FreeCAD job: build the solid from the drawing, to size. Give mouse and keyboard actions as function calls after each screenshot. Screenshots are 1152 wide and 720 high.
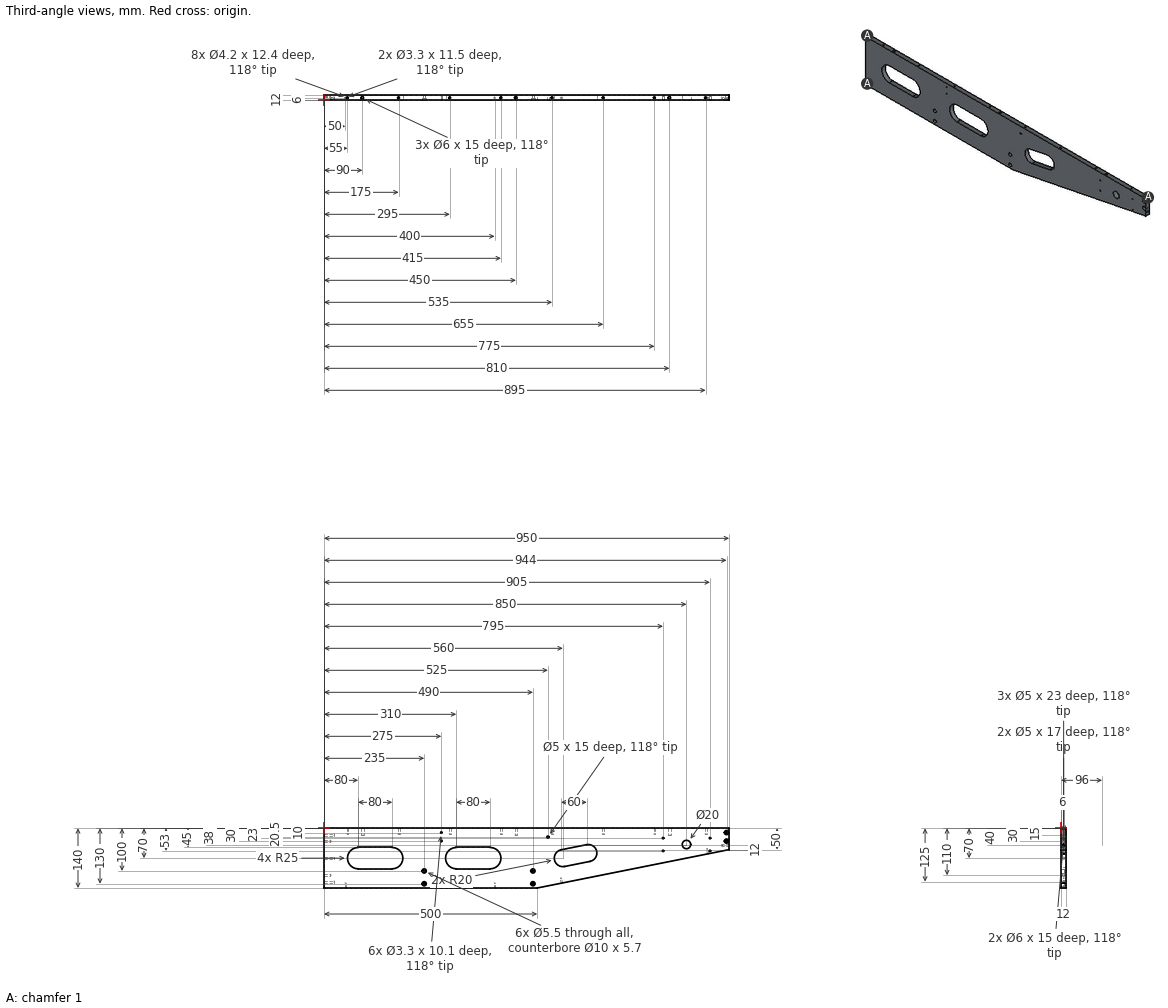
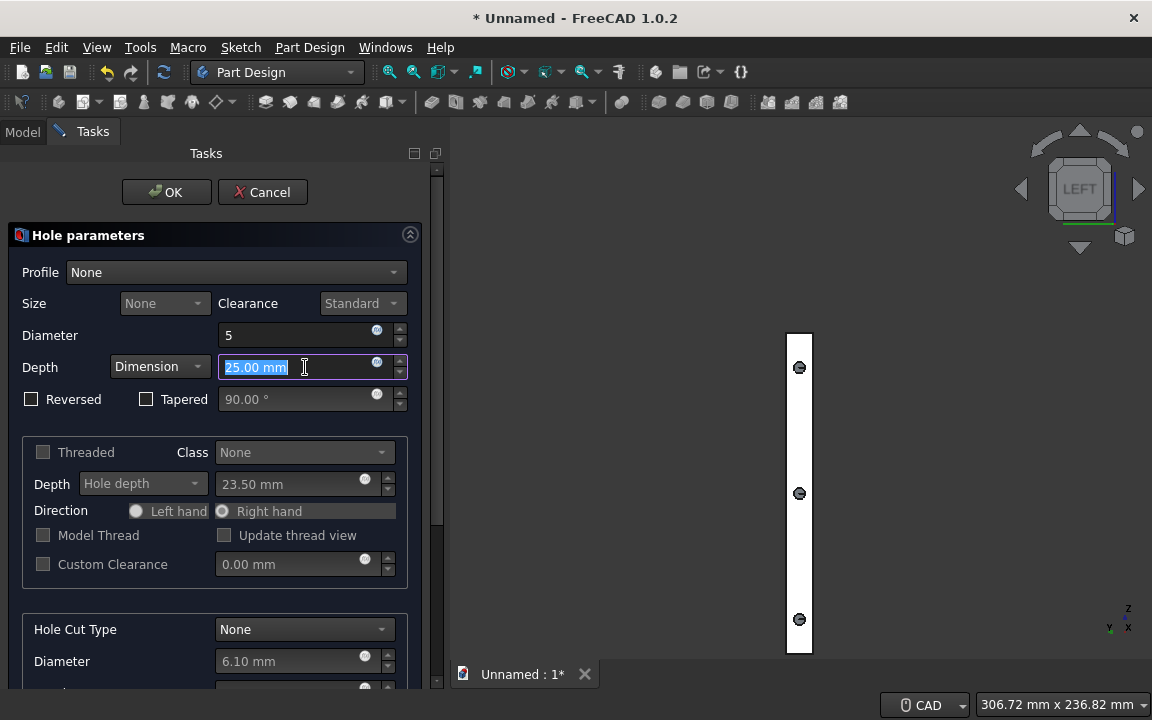
text(23)
key(Tab)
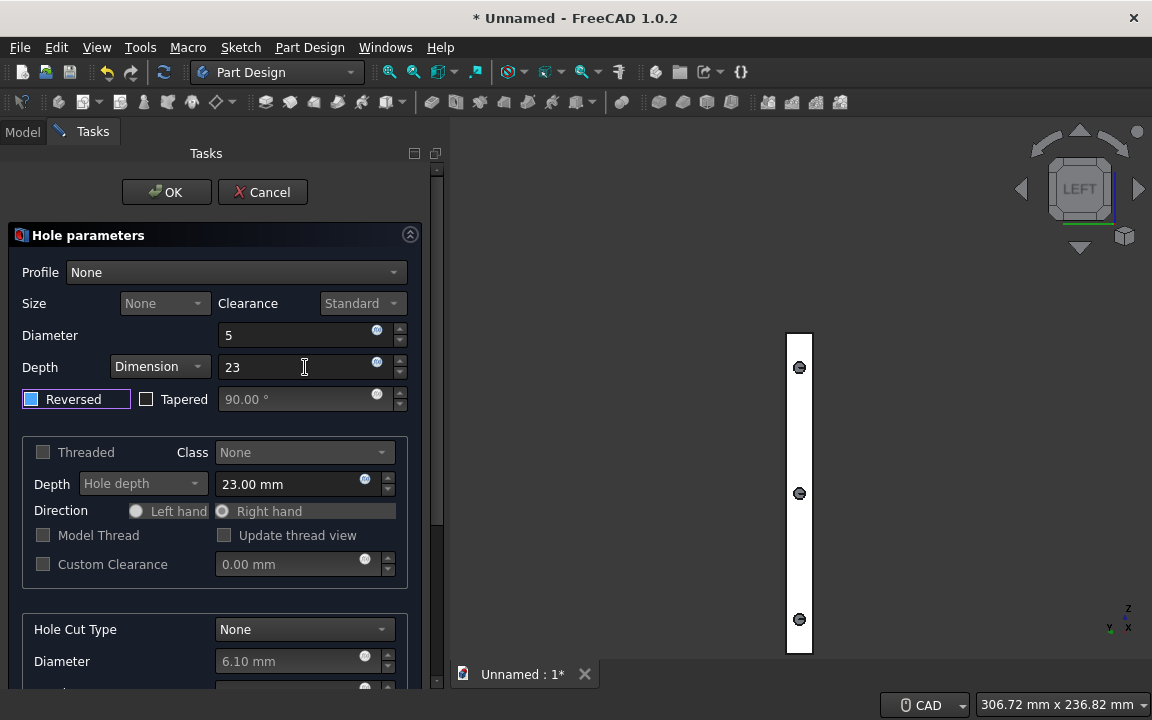
click(167, 192)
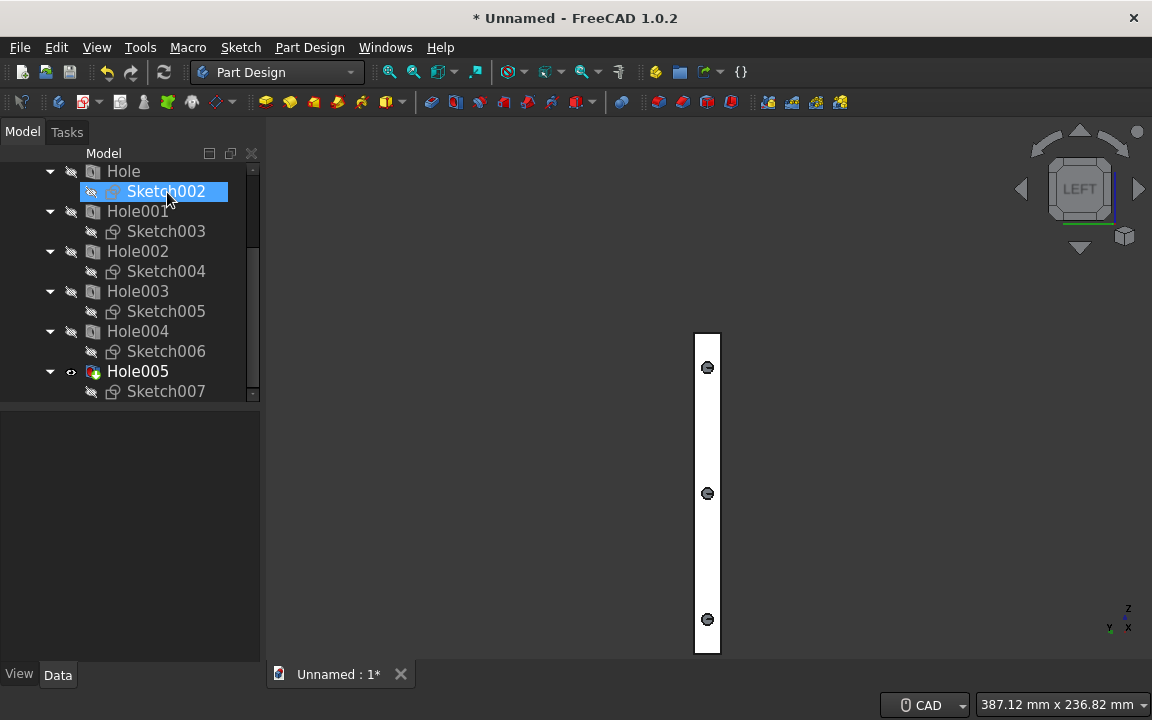
click(707, 401)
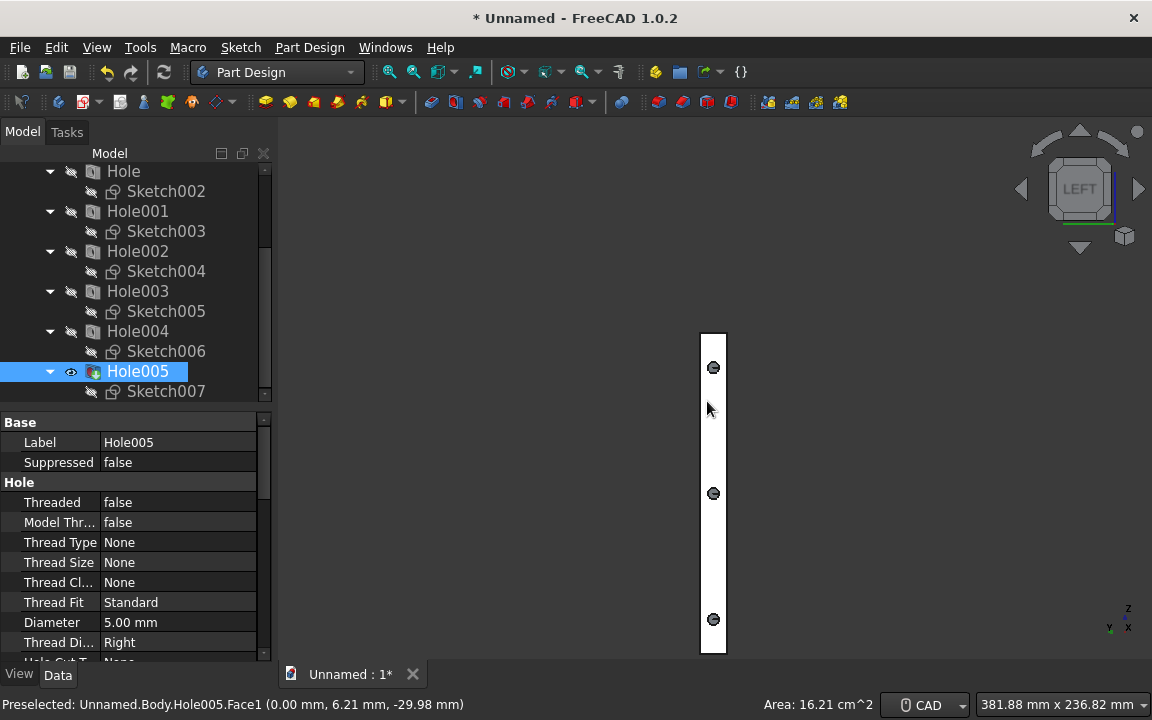
click(84, 102)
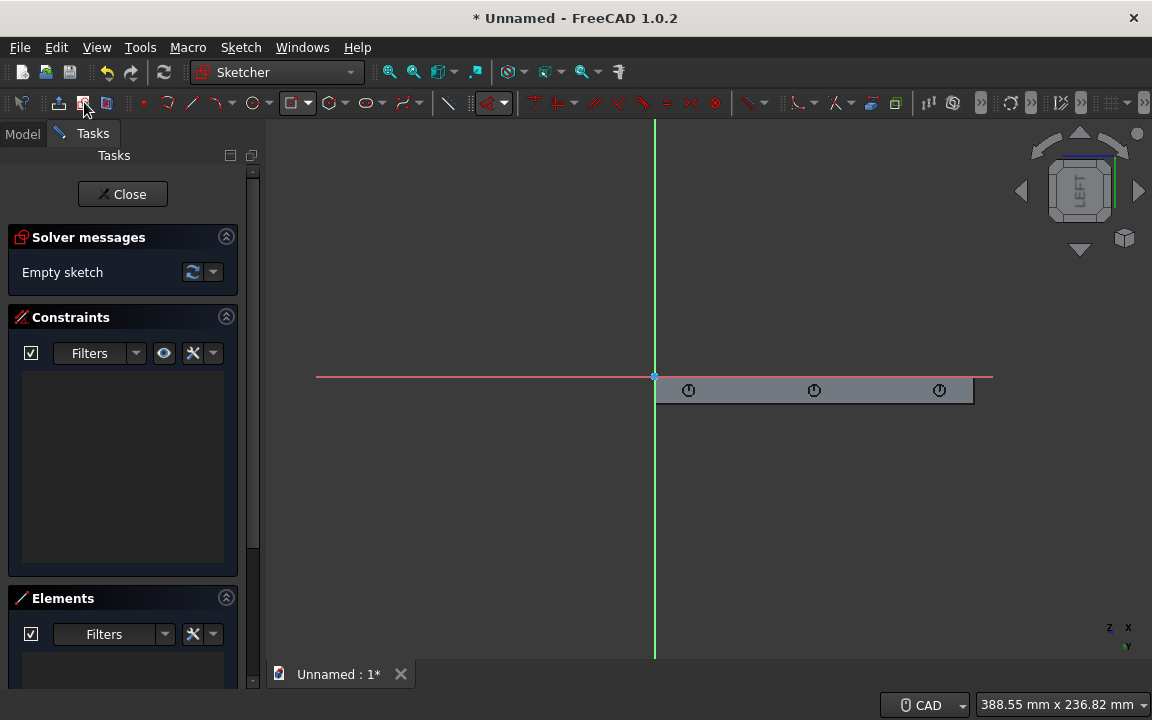
scroll(957, 385, up, 3)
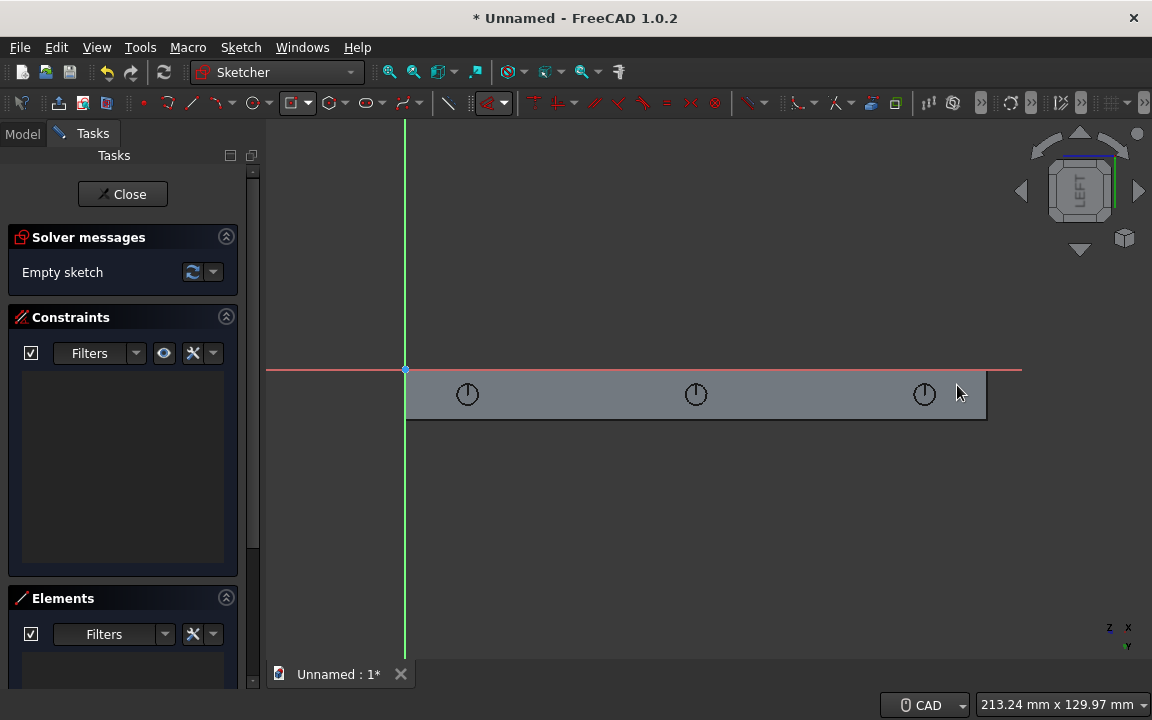
key(g)
key(c)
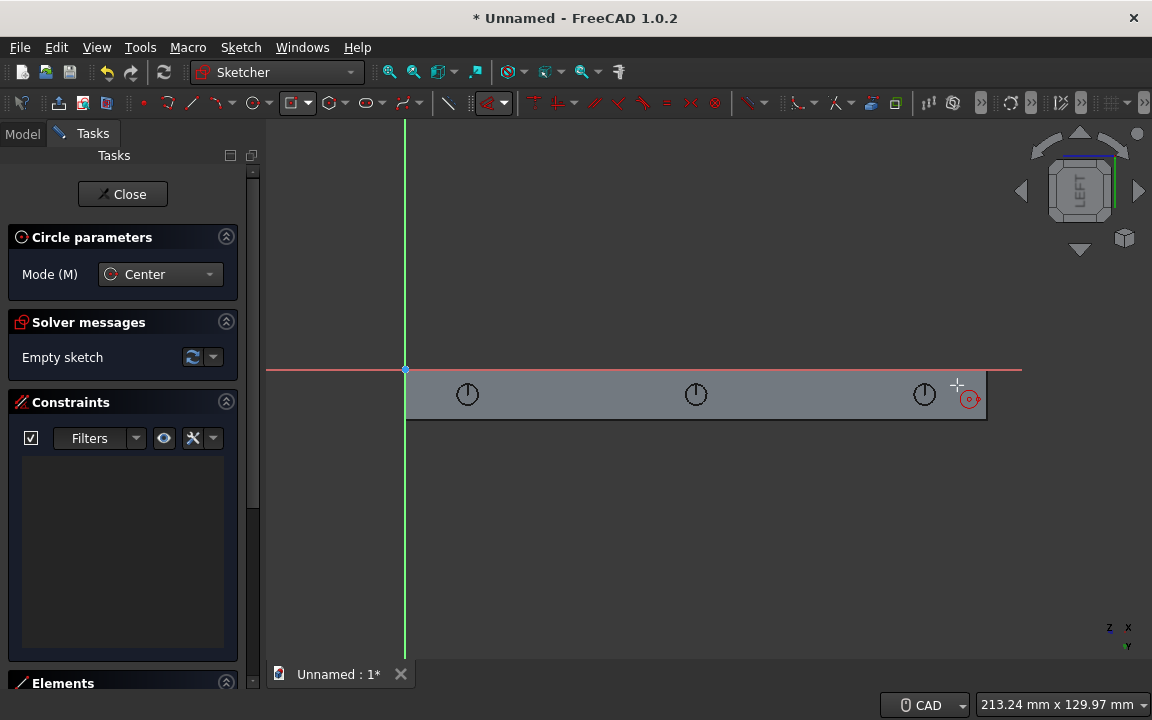
scroll(530, 395, up, 3)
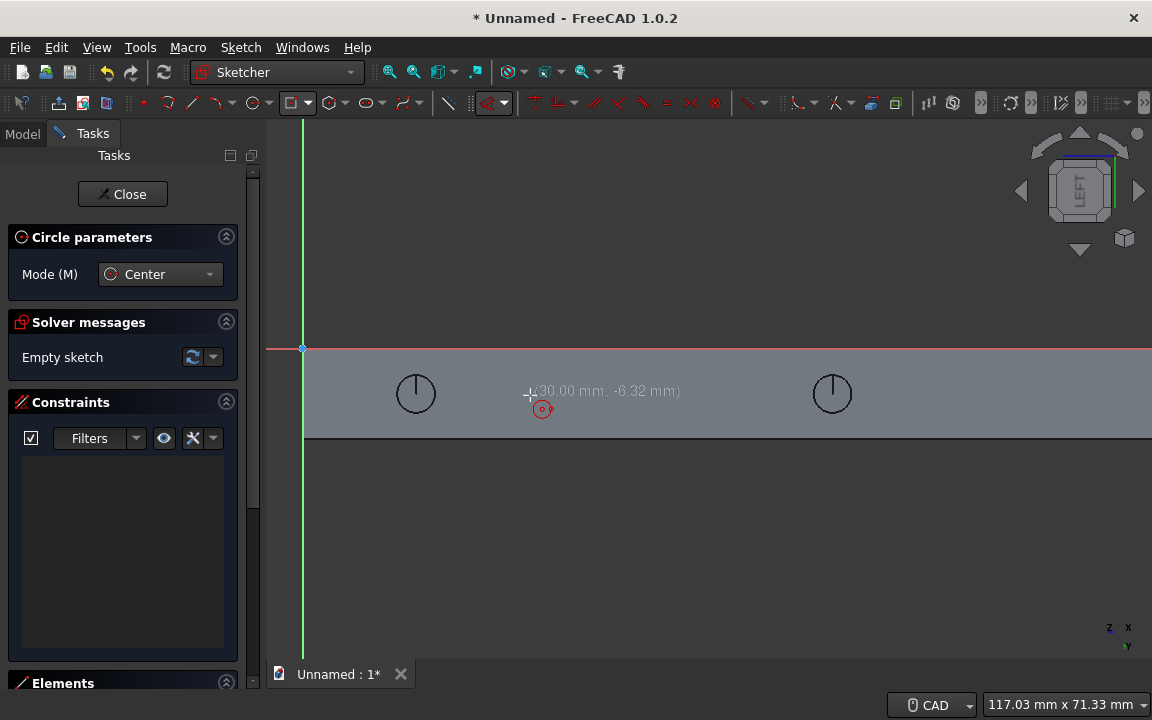
click(530, 394)
move(546, 378)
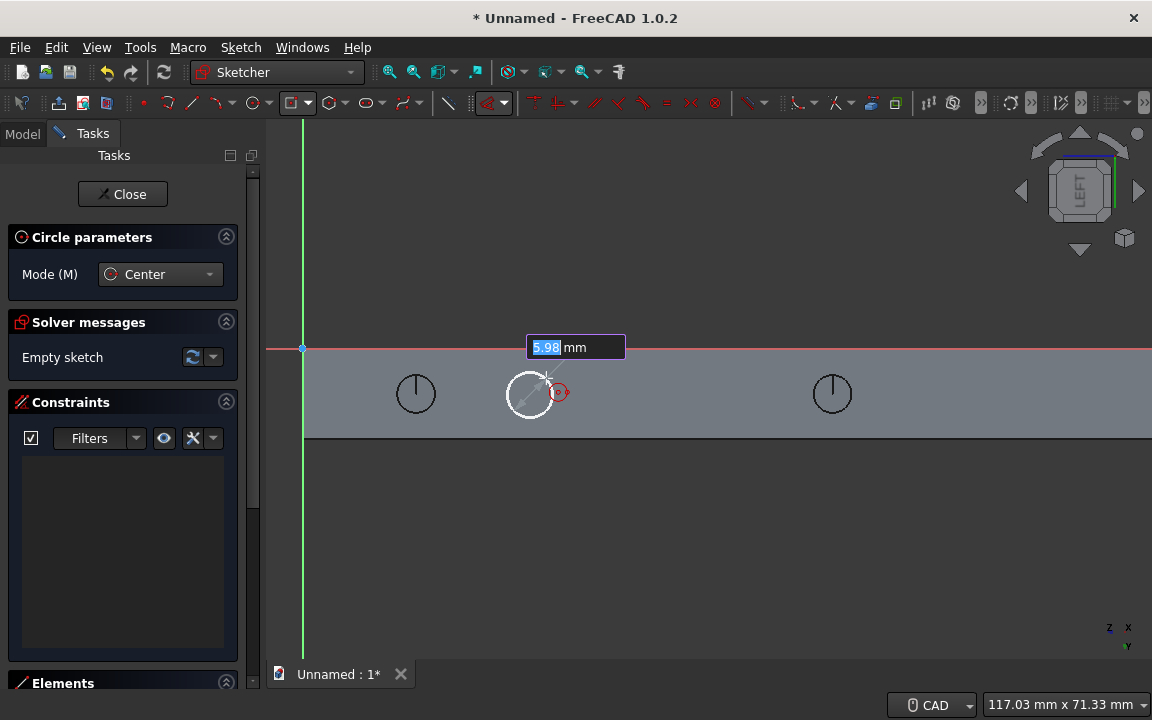
text(6)
key(Return)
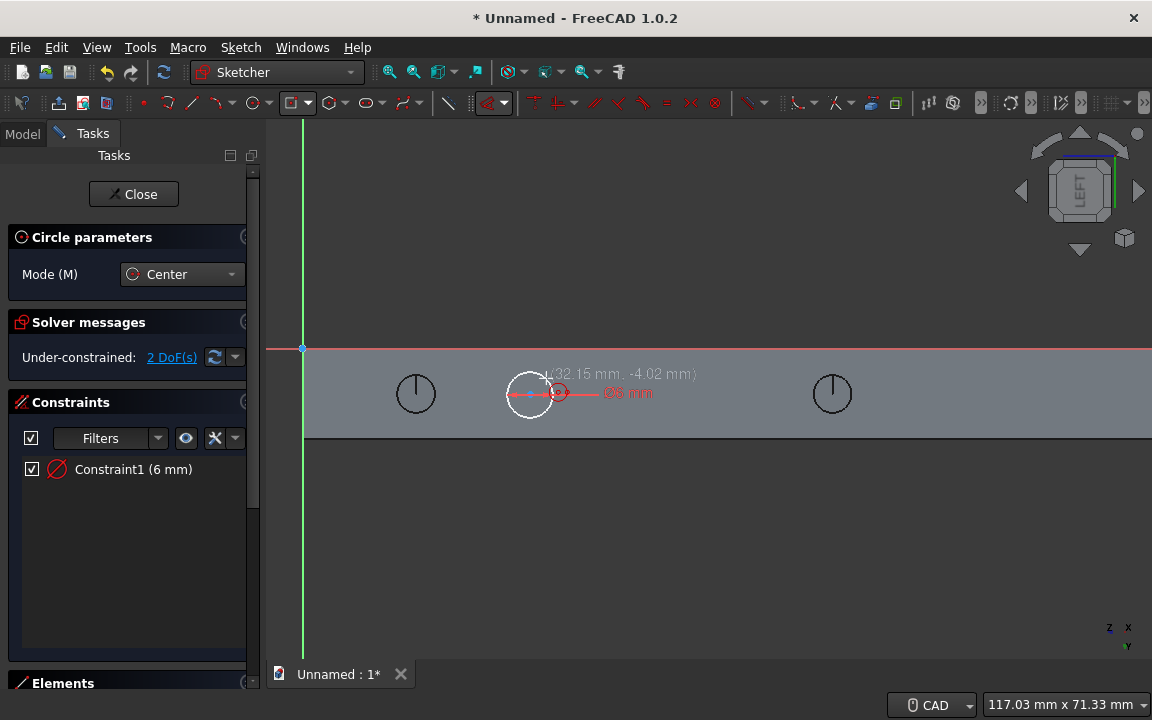
scroll(531, 397, down, 3)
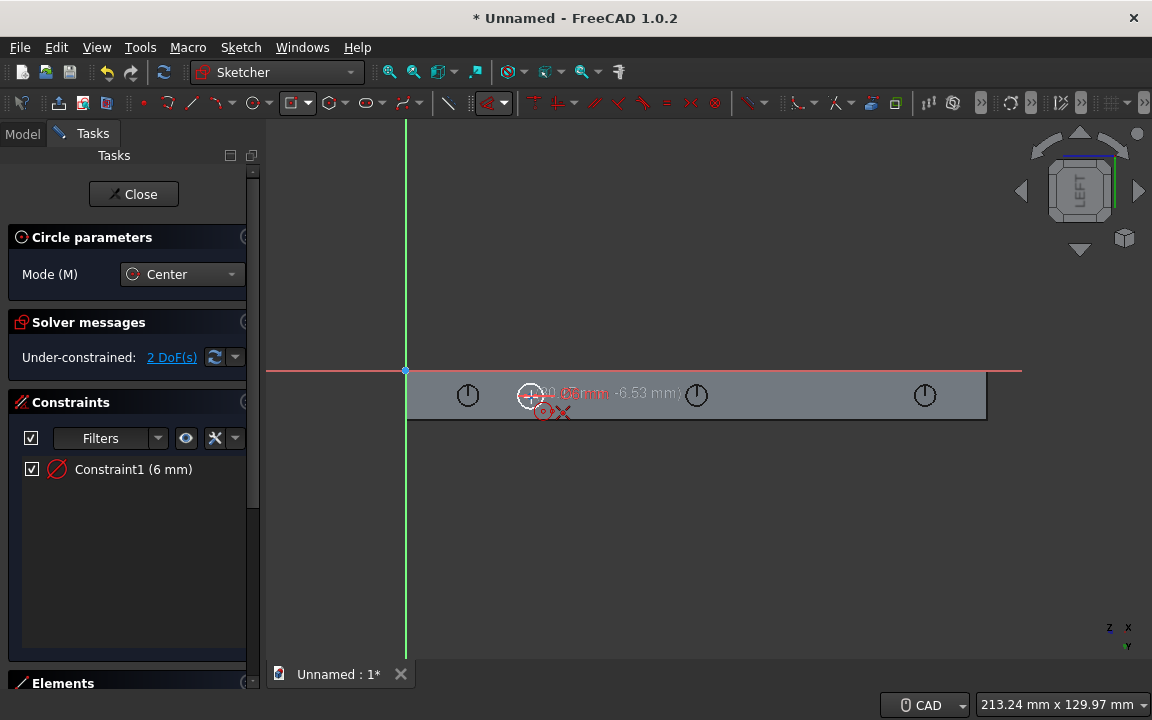
scroll(863, 396, up, 3)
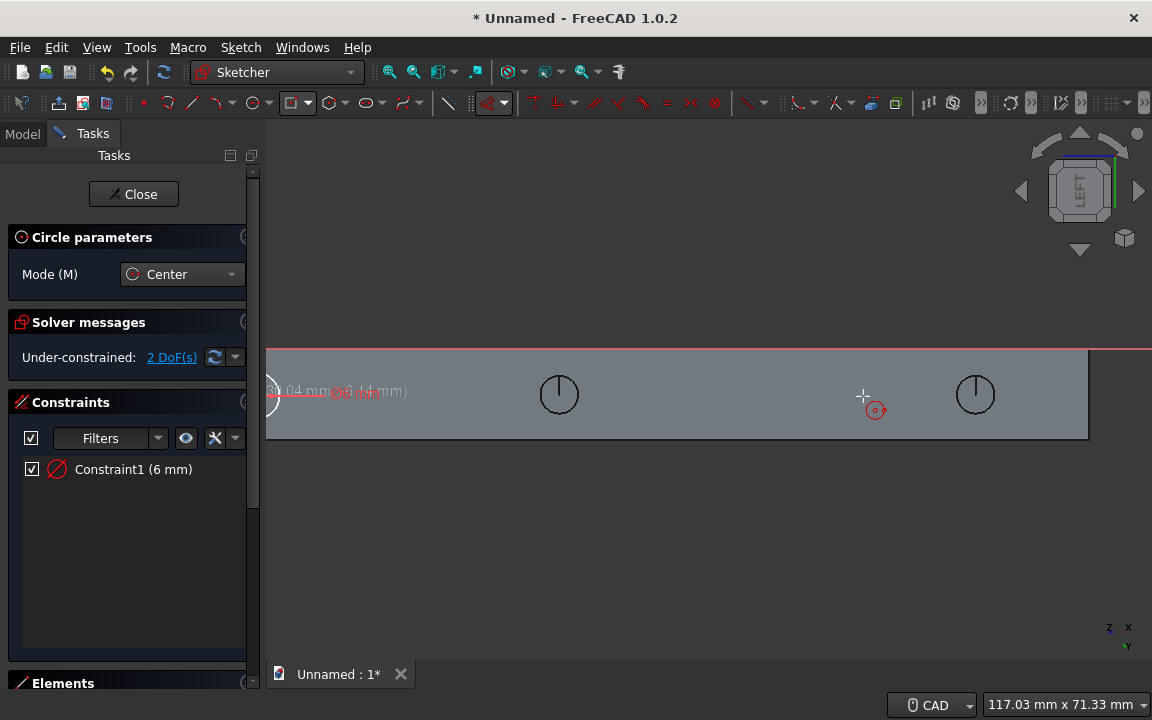
click(862, 395)
move(878, 379)